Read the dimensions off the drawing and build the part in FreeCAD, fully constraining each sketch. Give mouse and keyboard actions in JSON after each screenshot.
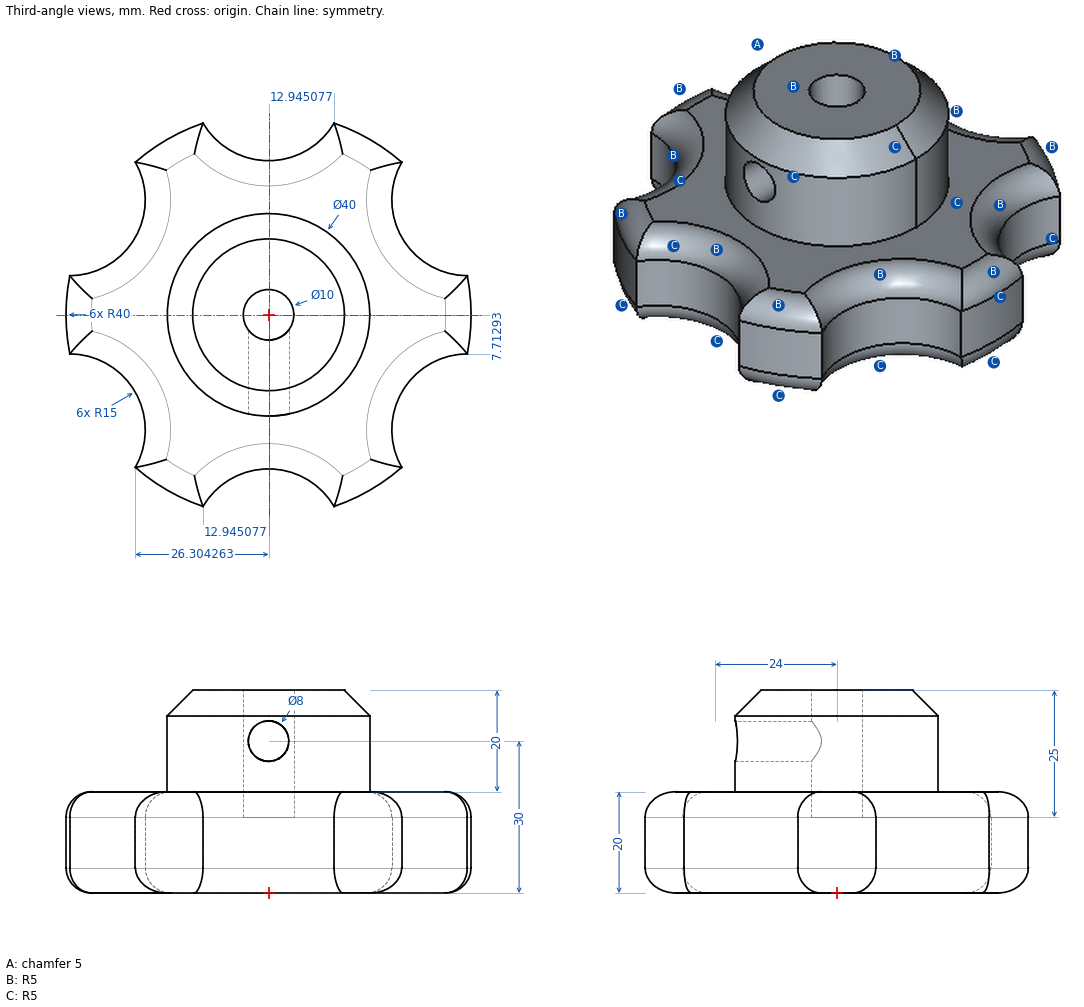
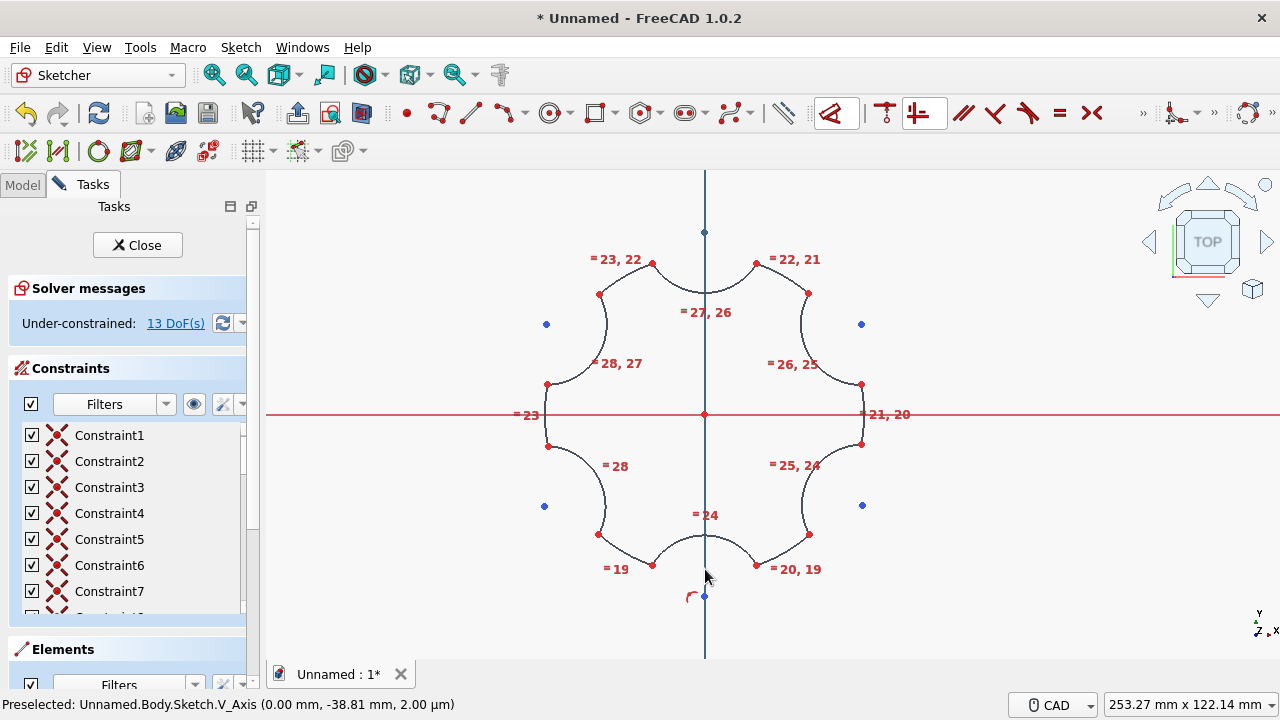
{"action": "left_click", "coordinate": [886, 114]}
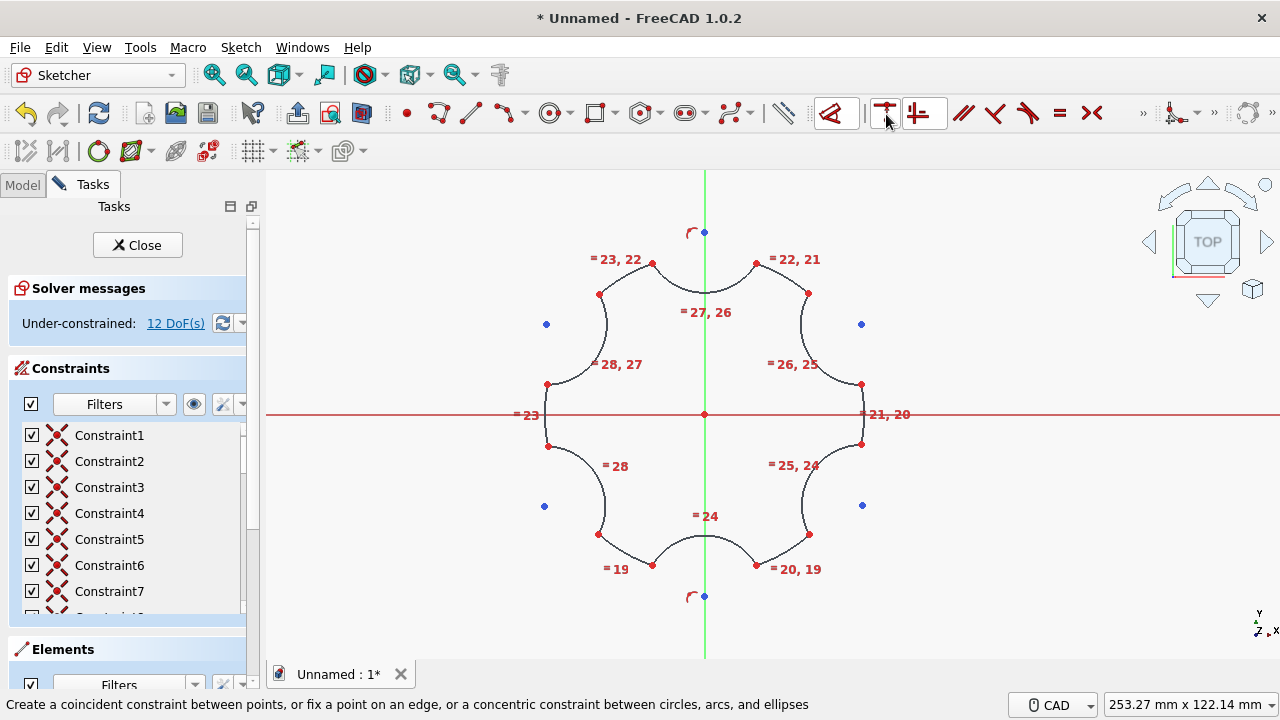
{"action": "left_click", "coordinate": [862, 505]}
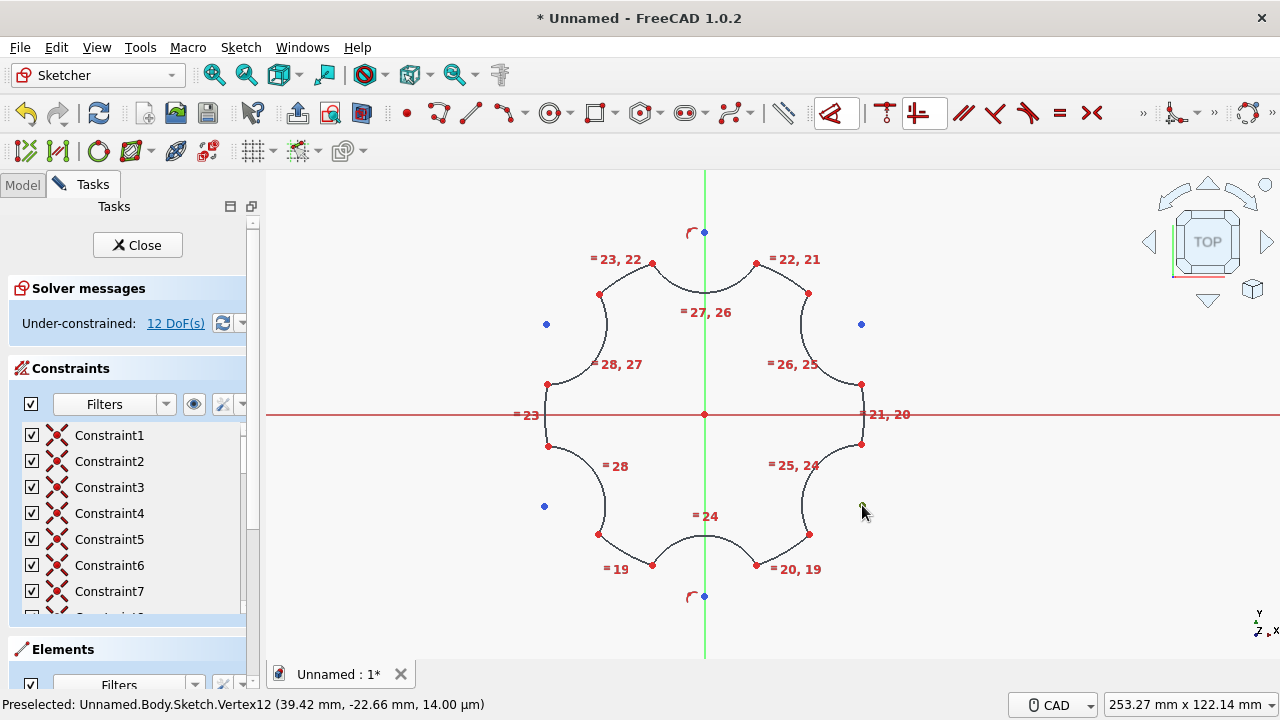
{"action": "left_click", "coordinate": [861, 325]}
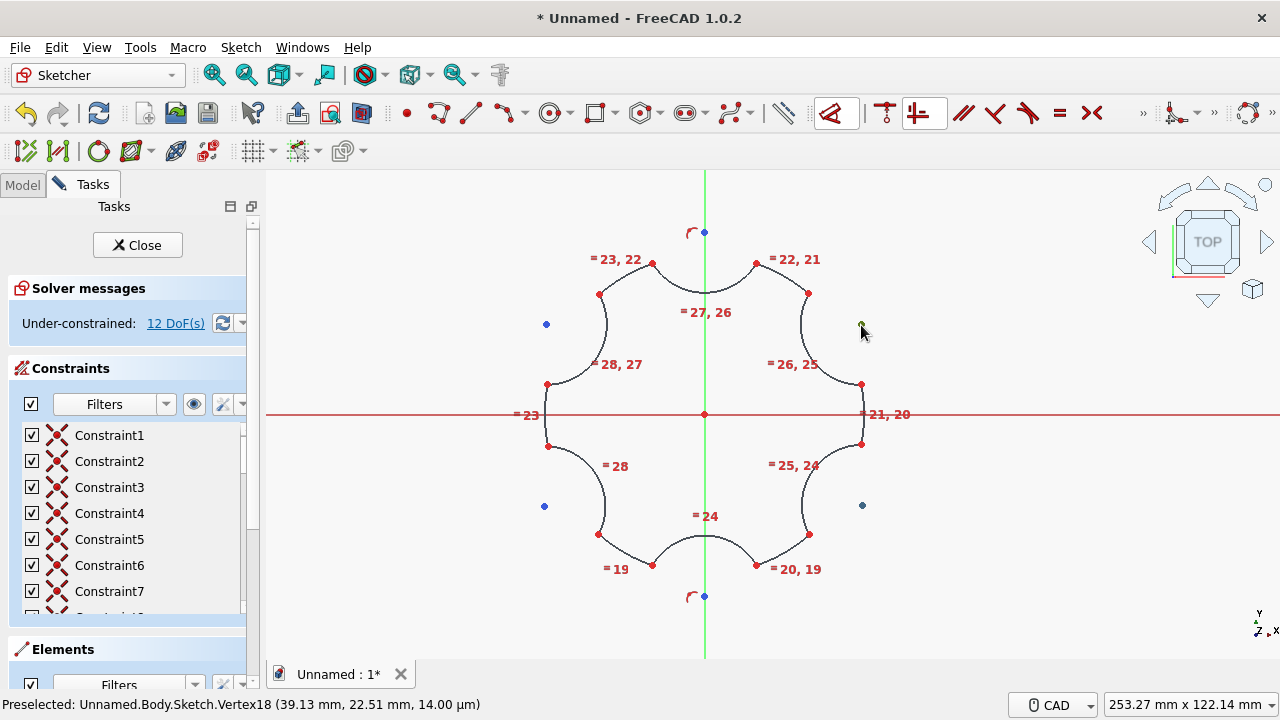
{"action": "left_click", "coordinate": [353, 415]}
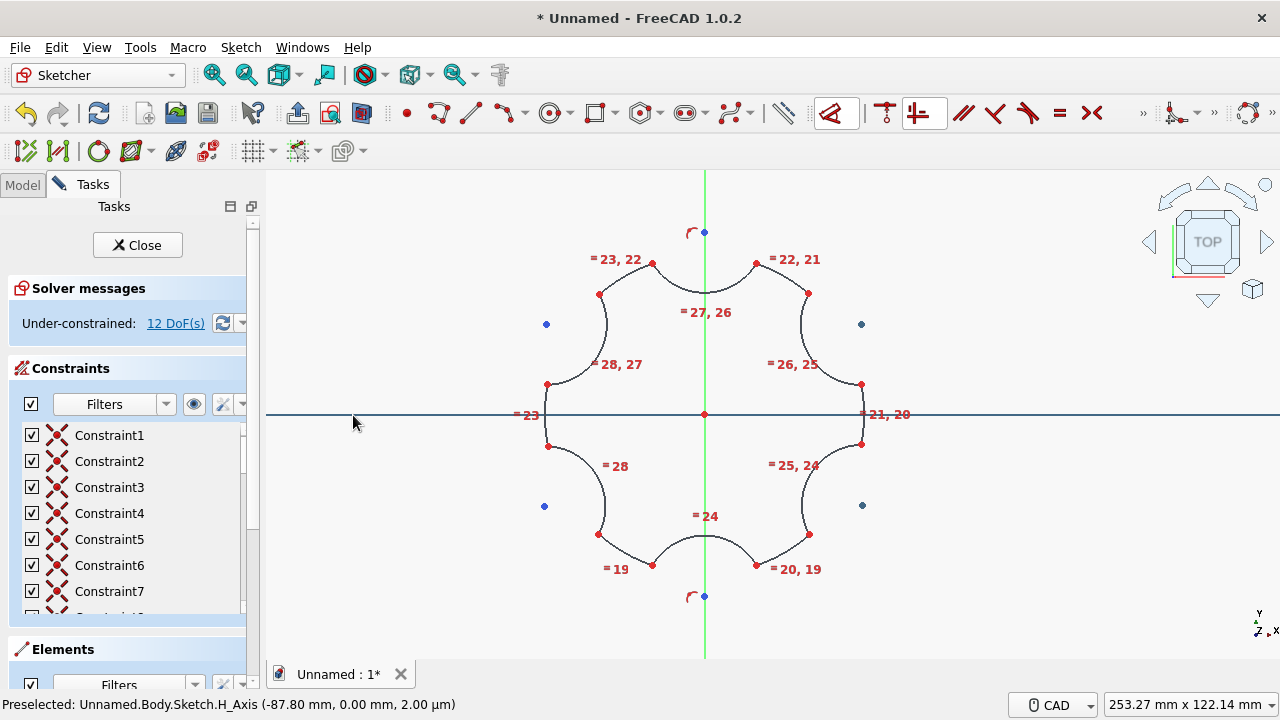
{"action": "left_click", "coordinate": [1092, 114]}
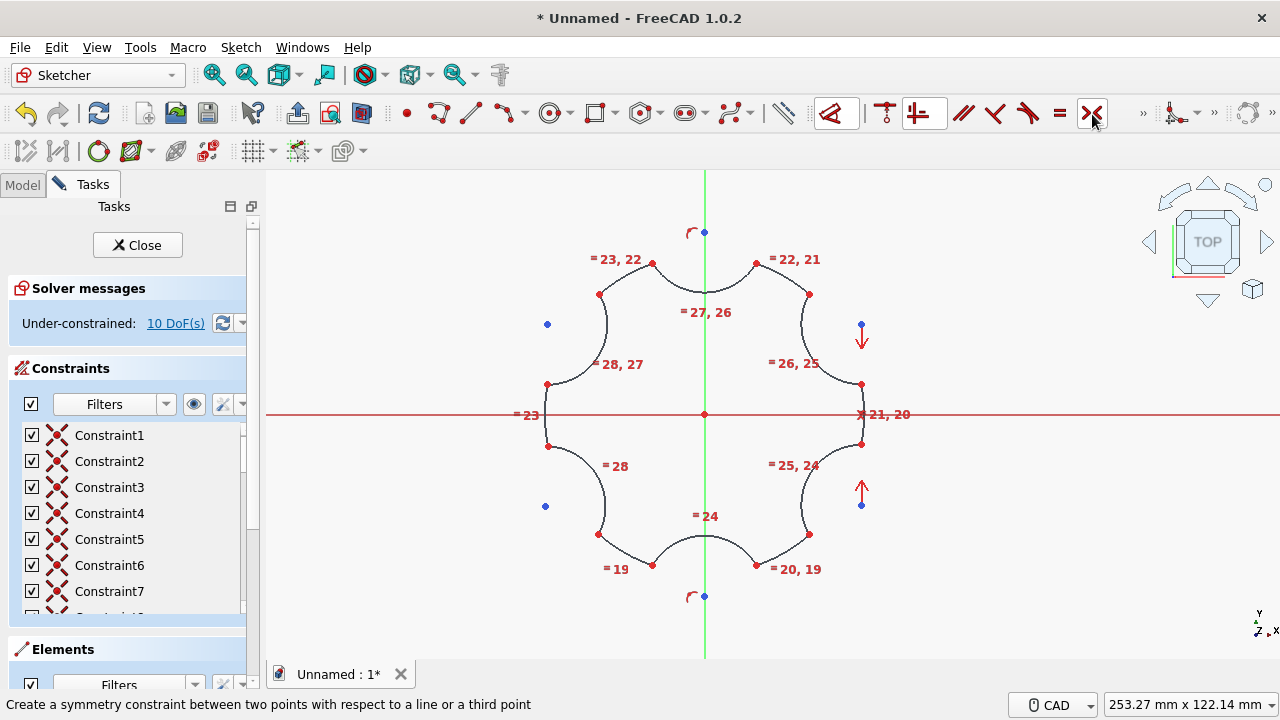
{"action": "left_click", "coordinate": [862, 324]}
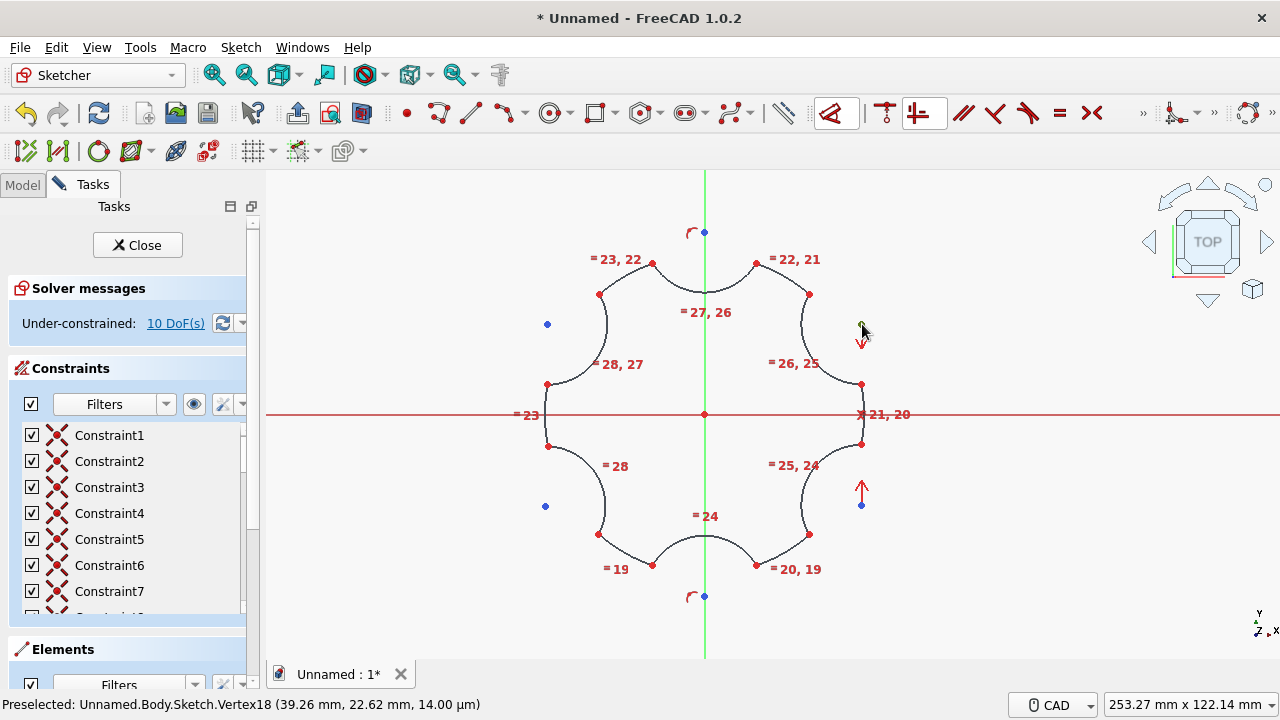
{"action": "left_click", "coordinate": [547, 324]}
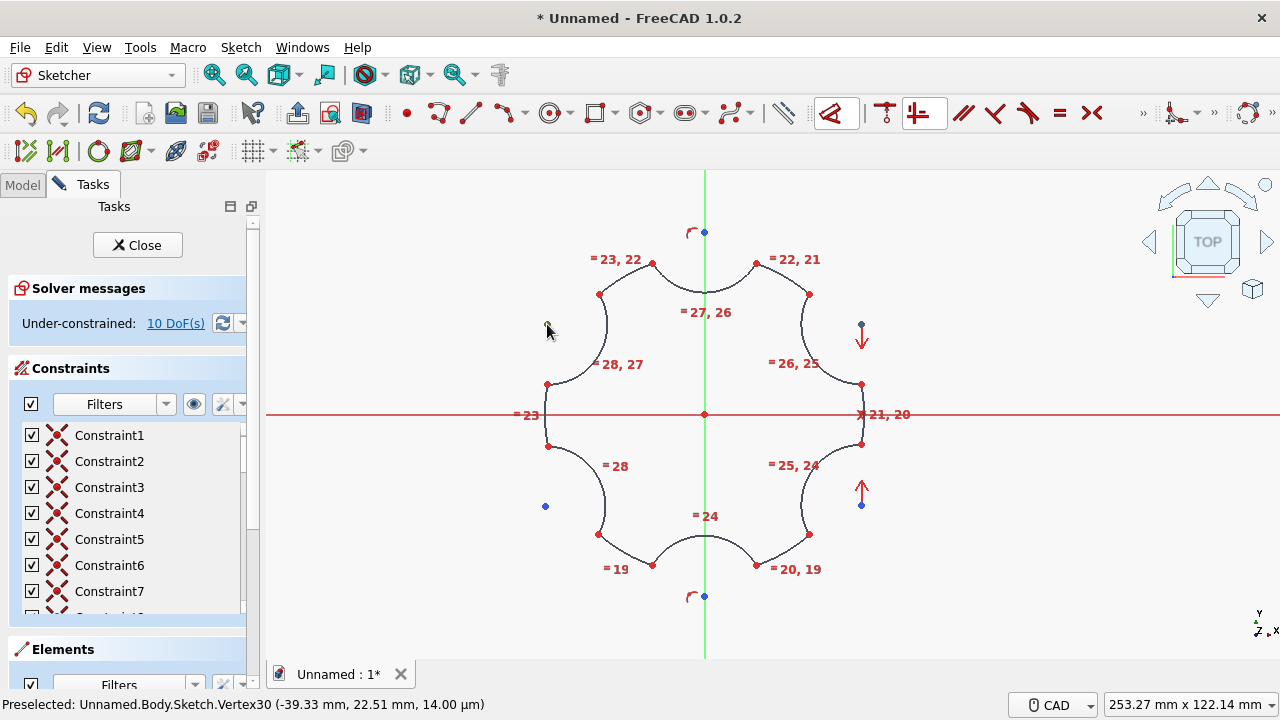
{"action": "left_click", "coordinate": [705, 569]}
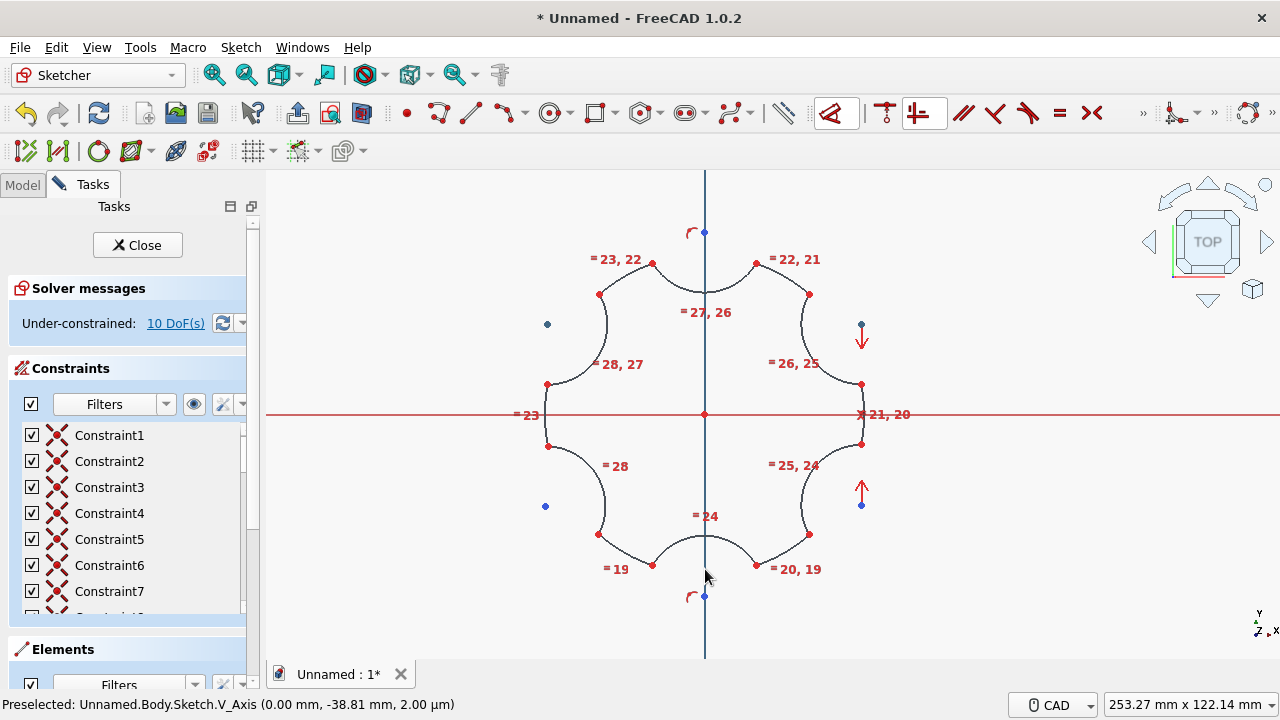
{"action": "left_click", "coordinate": [1092, 114]}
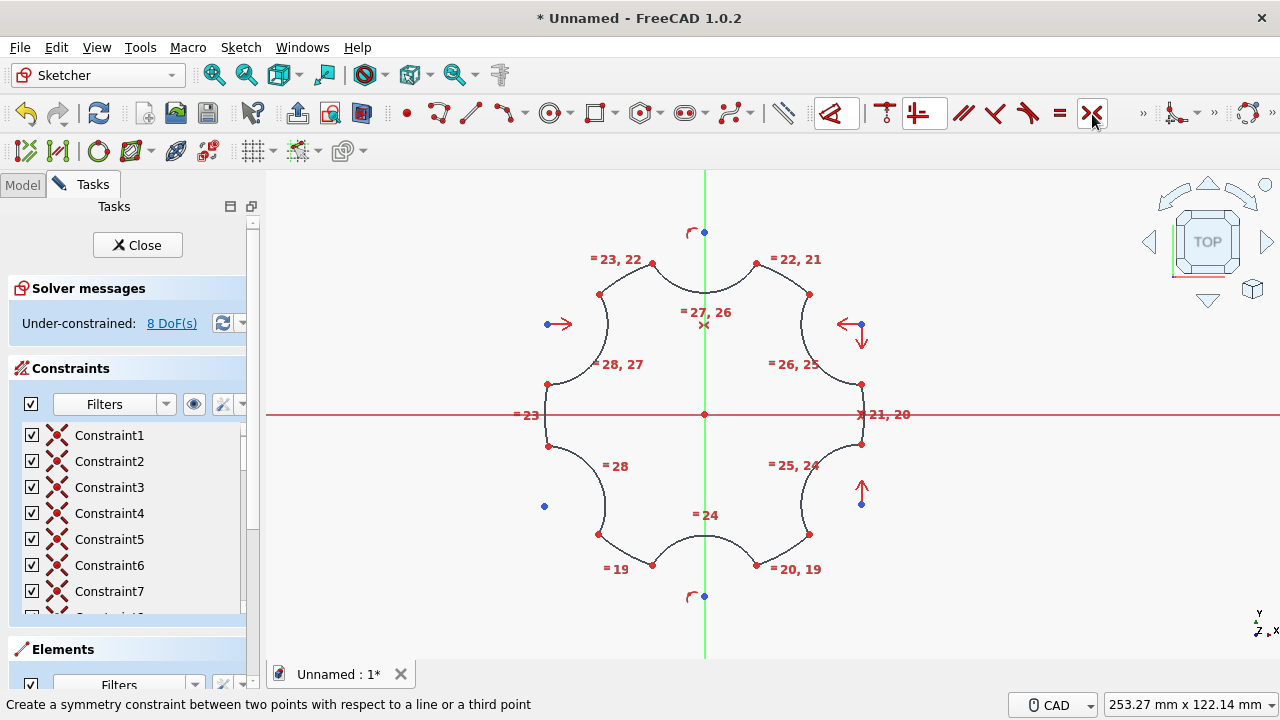
{"action": "left_click", "coordinate": [862, 505]}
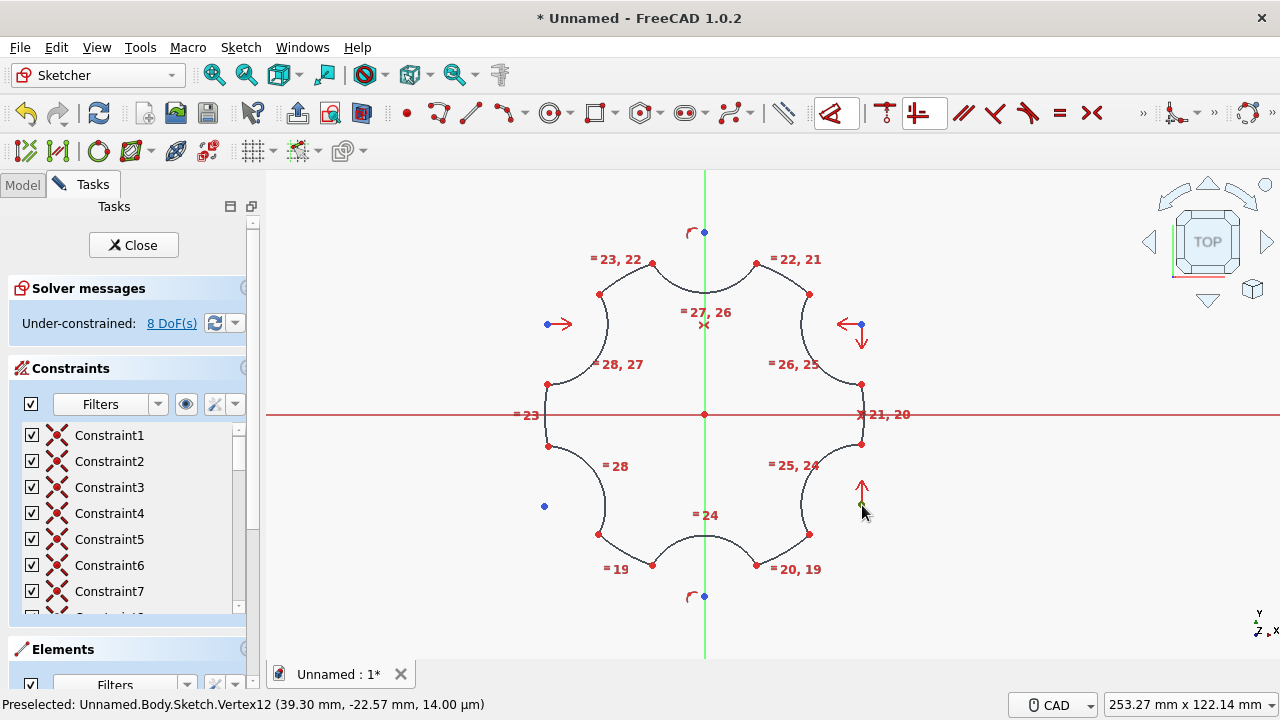
{"action": "left_click", "coordinate": [545, 507]}